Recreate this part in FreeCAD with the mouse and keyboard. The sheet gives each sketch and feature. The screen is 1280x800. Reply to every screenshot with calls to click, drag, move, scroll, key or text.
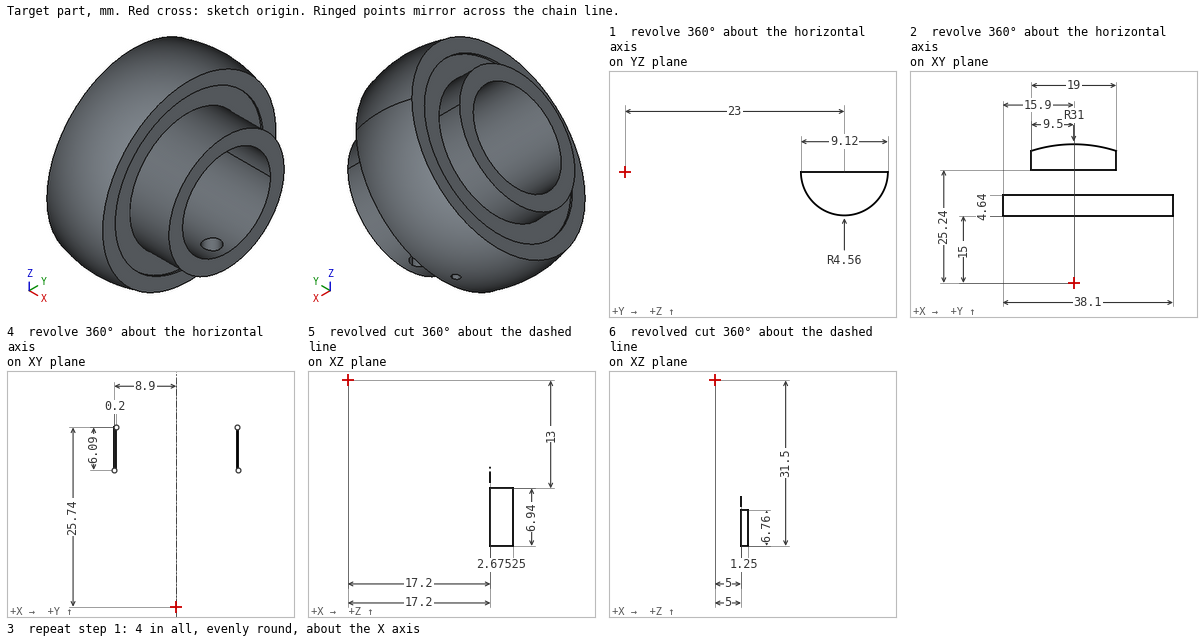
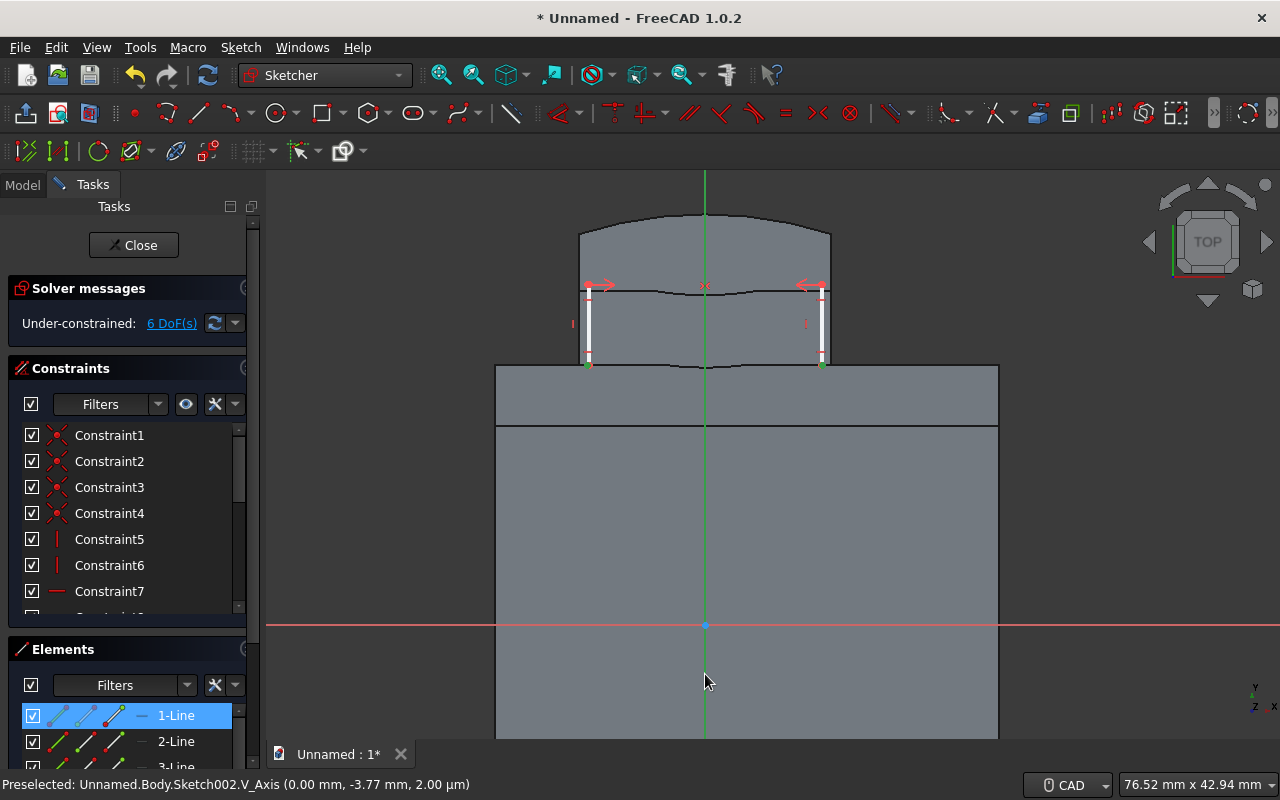
click(818, 114)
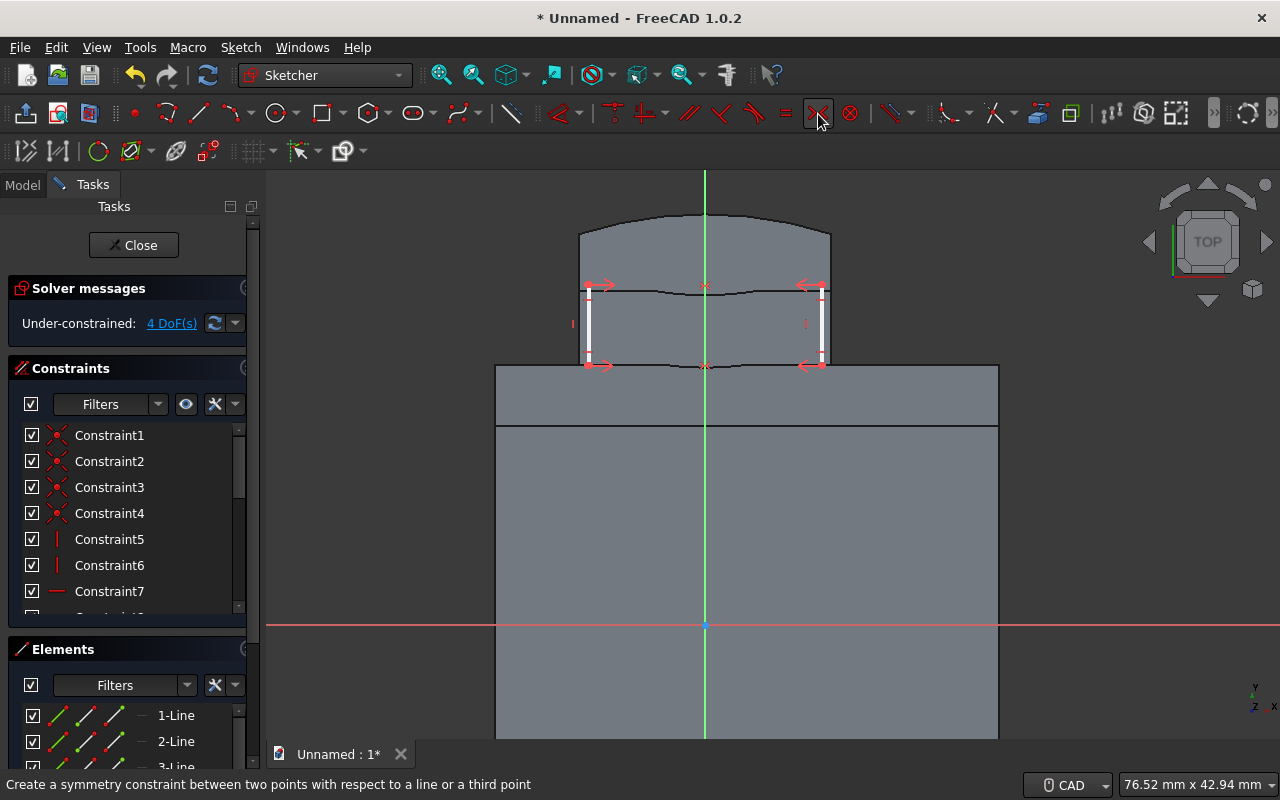
click(558, 114)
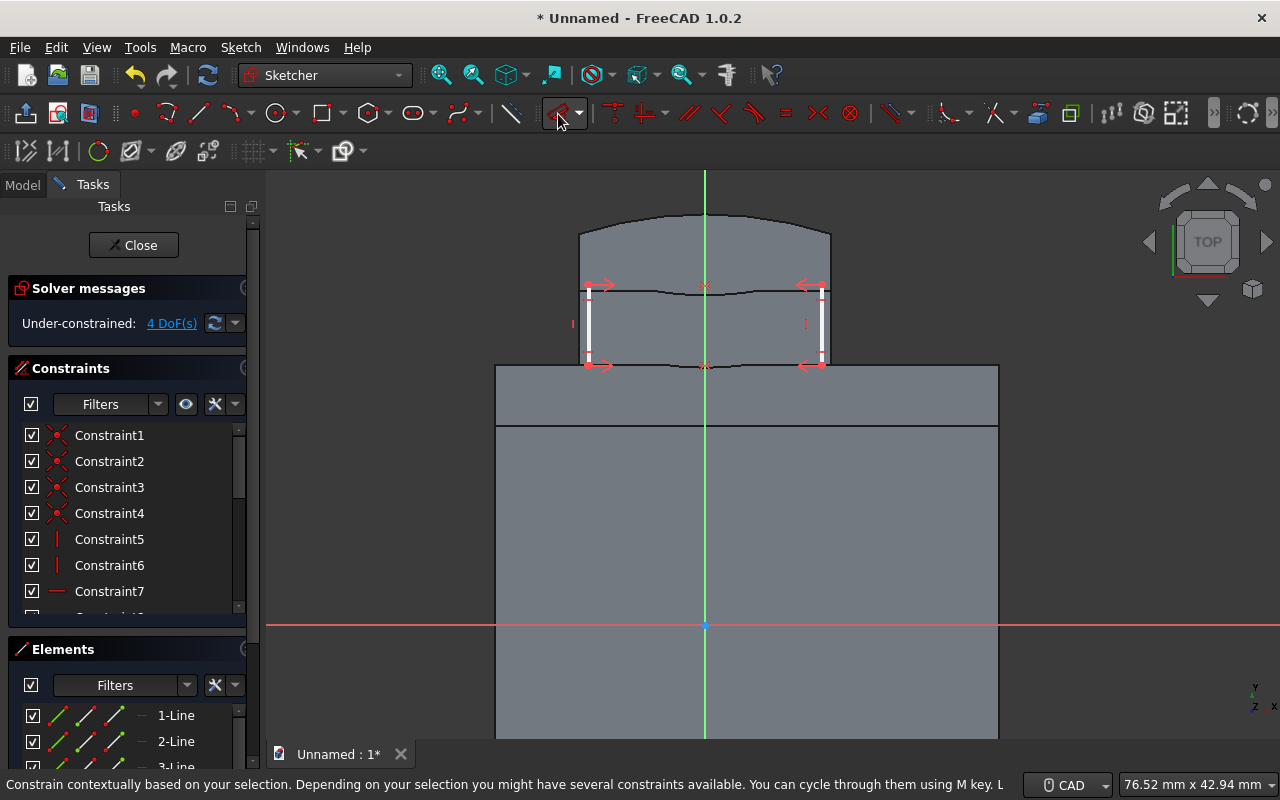
scroll(589, 366, up, 14)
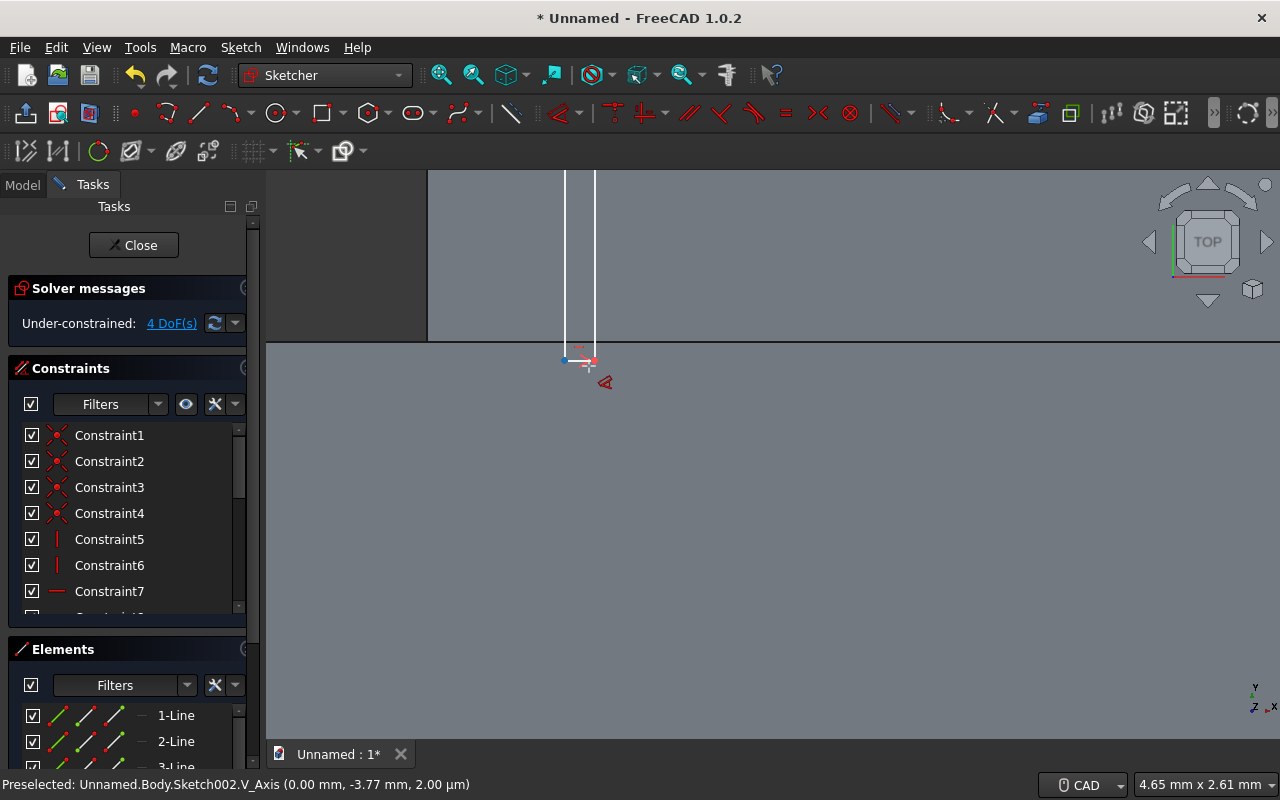
click(580, 361)
click(580, 327)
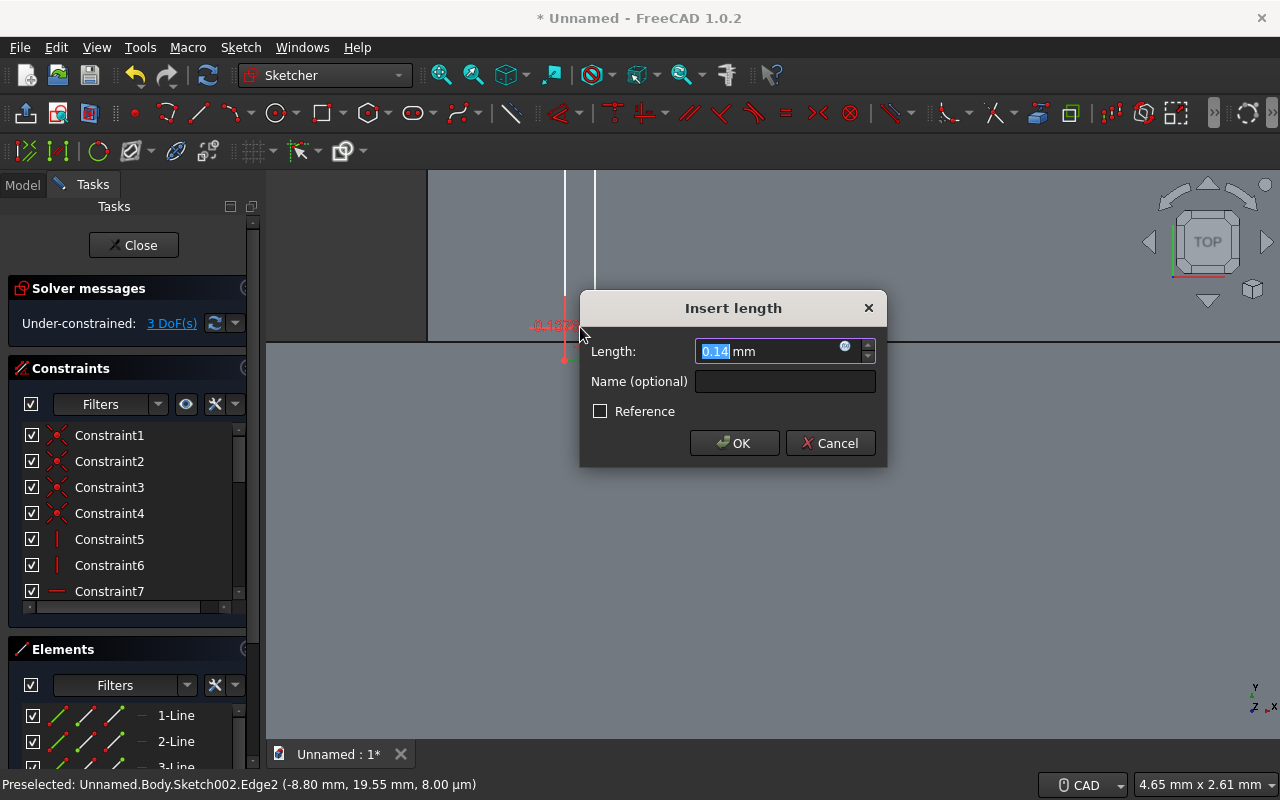
text(0.2)
key(Return)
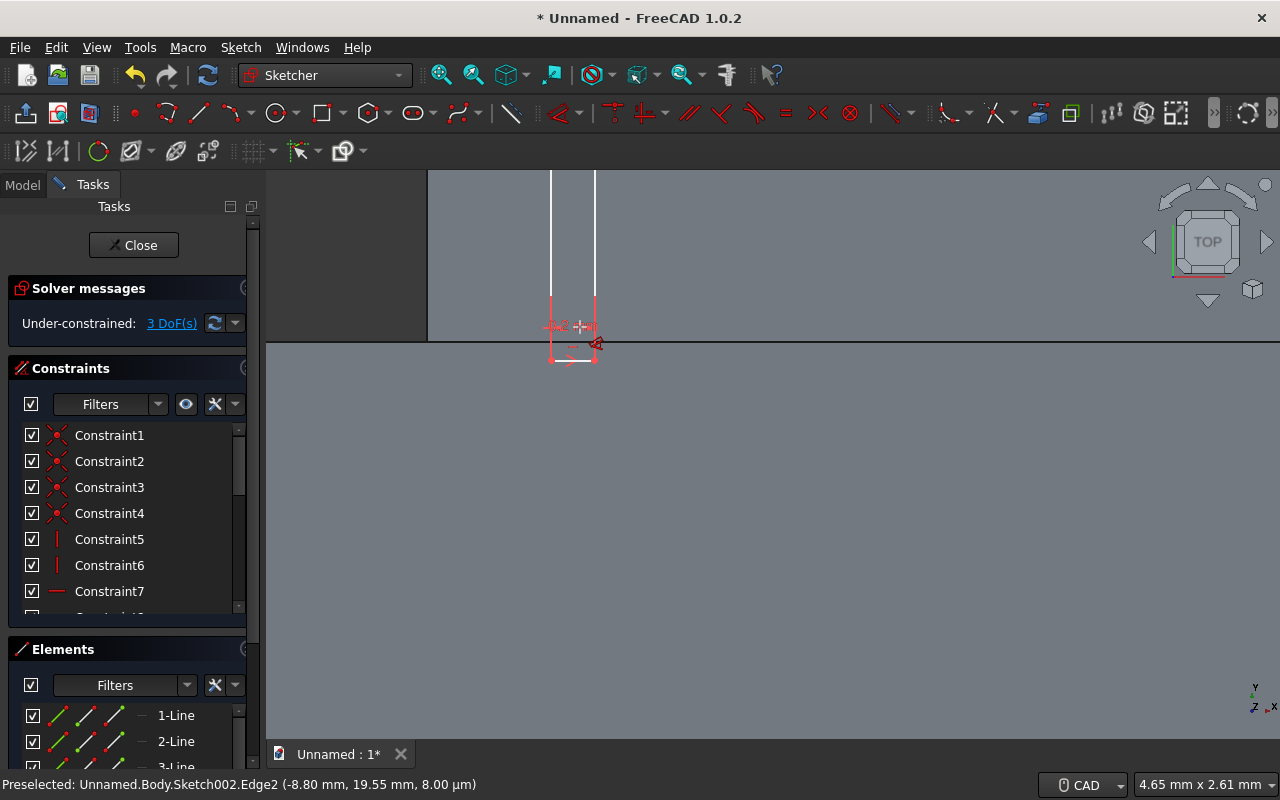
scroll(588, 366, down, 14)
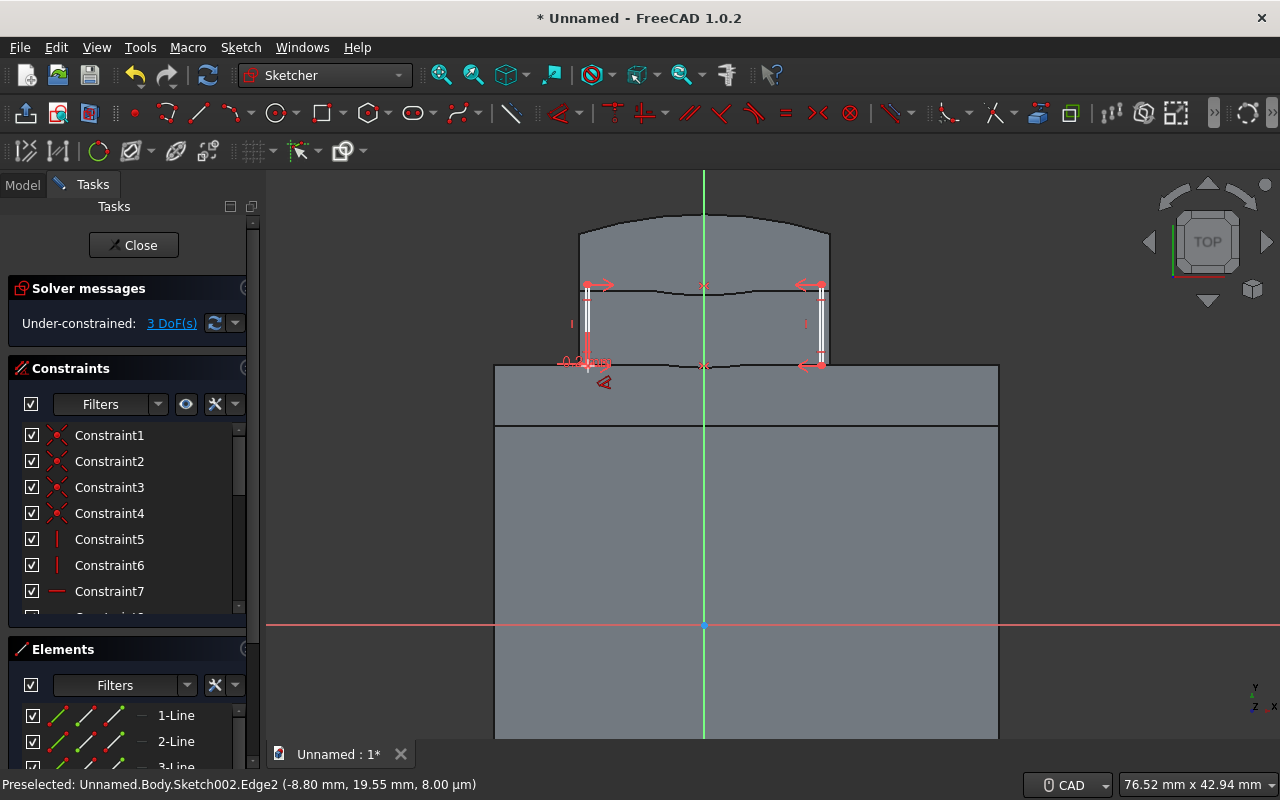
scroll(586, 309, up, 9)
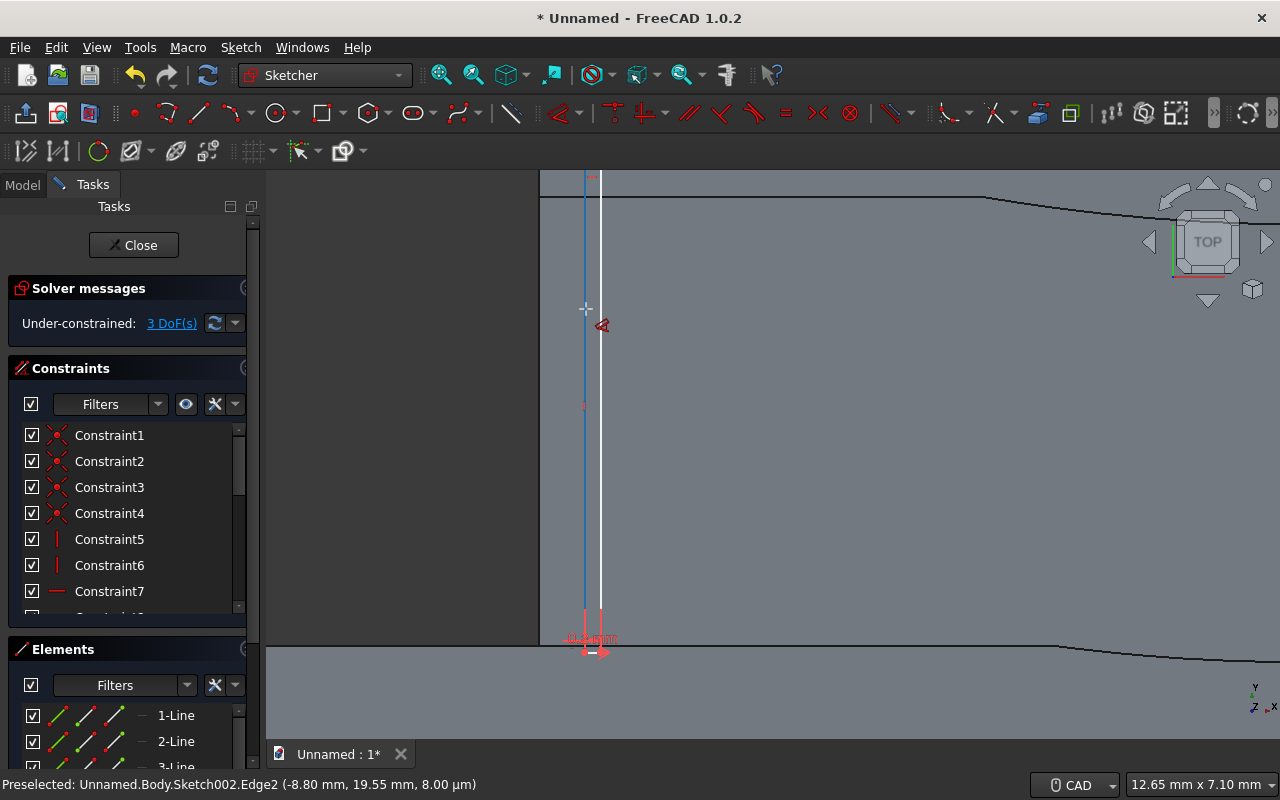
click(585, 310)
click(551, 425)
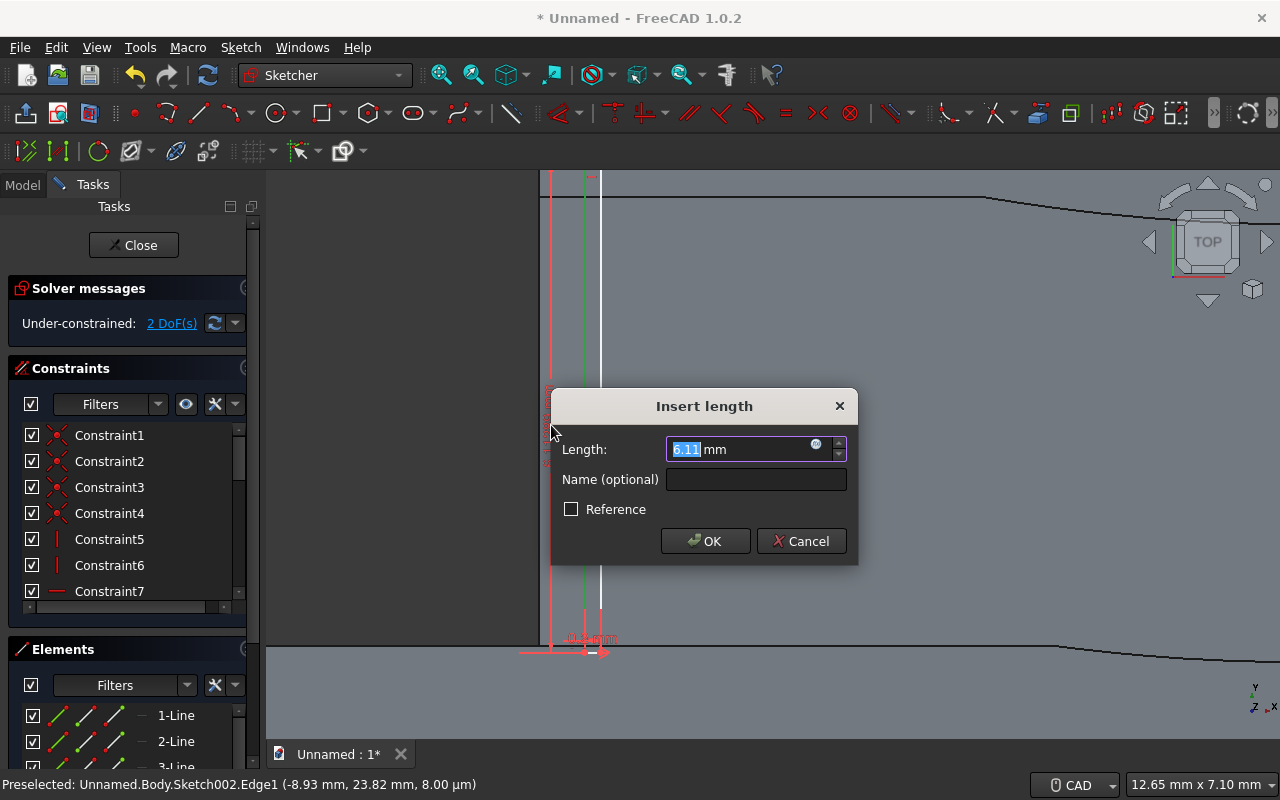
text(6.09)
key(Return)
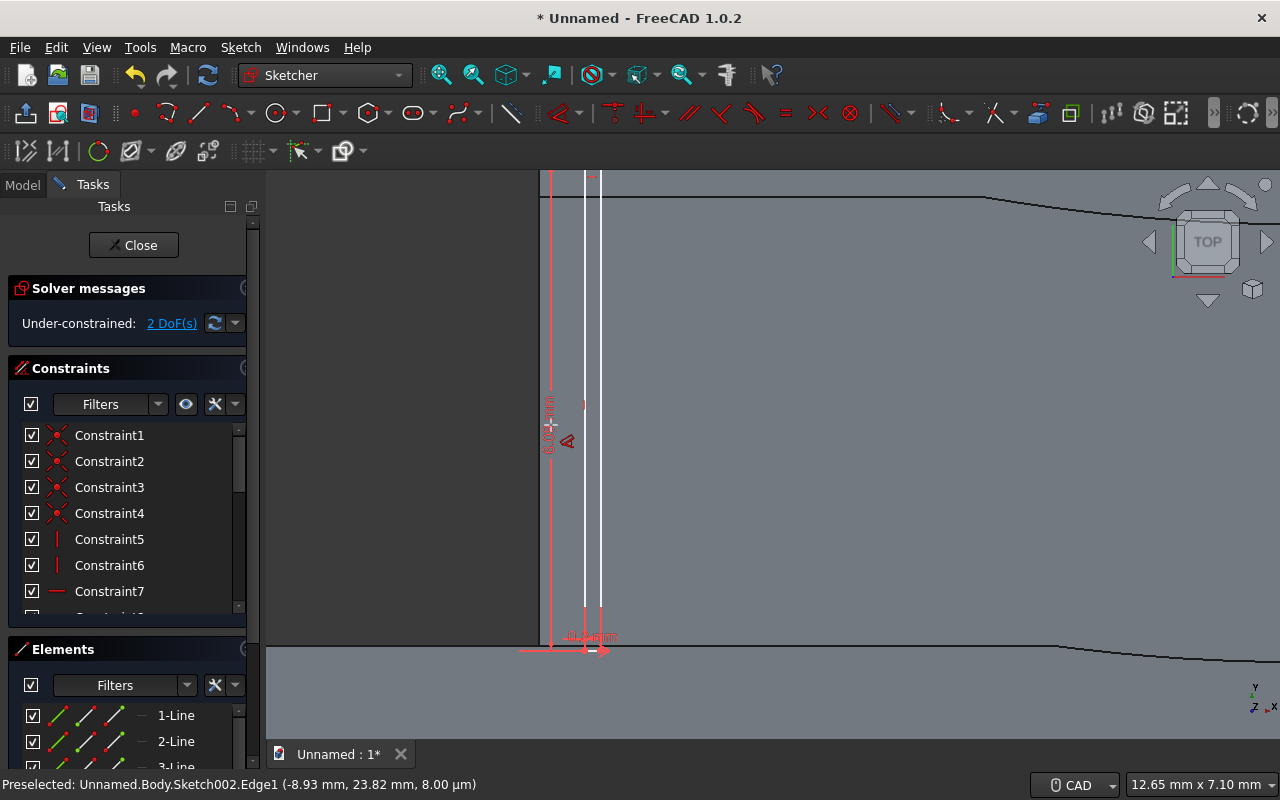
scroll(586, 309, down, 9)